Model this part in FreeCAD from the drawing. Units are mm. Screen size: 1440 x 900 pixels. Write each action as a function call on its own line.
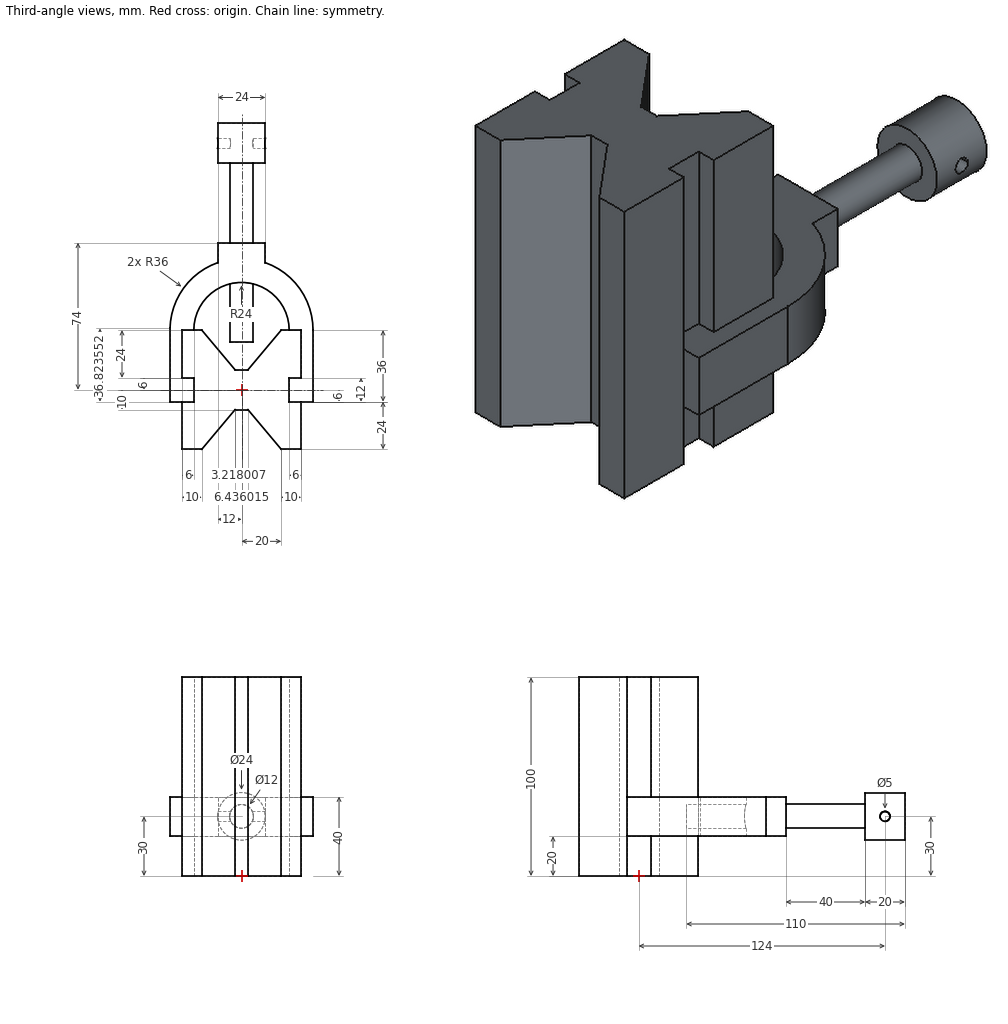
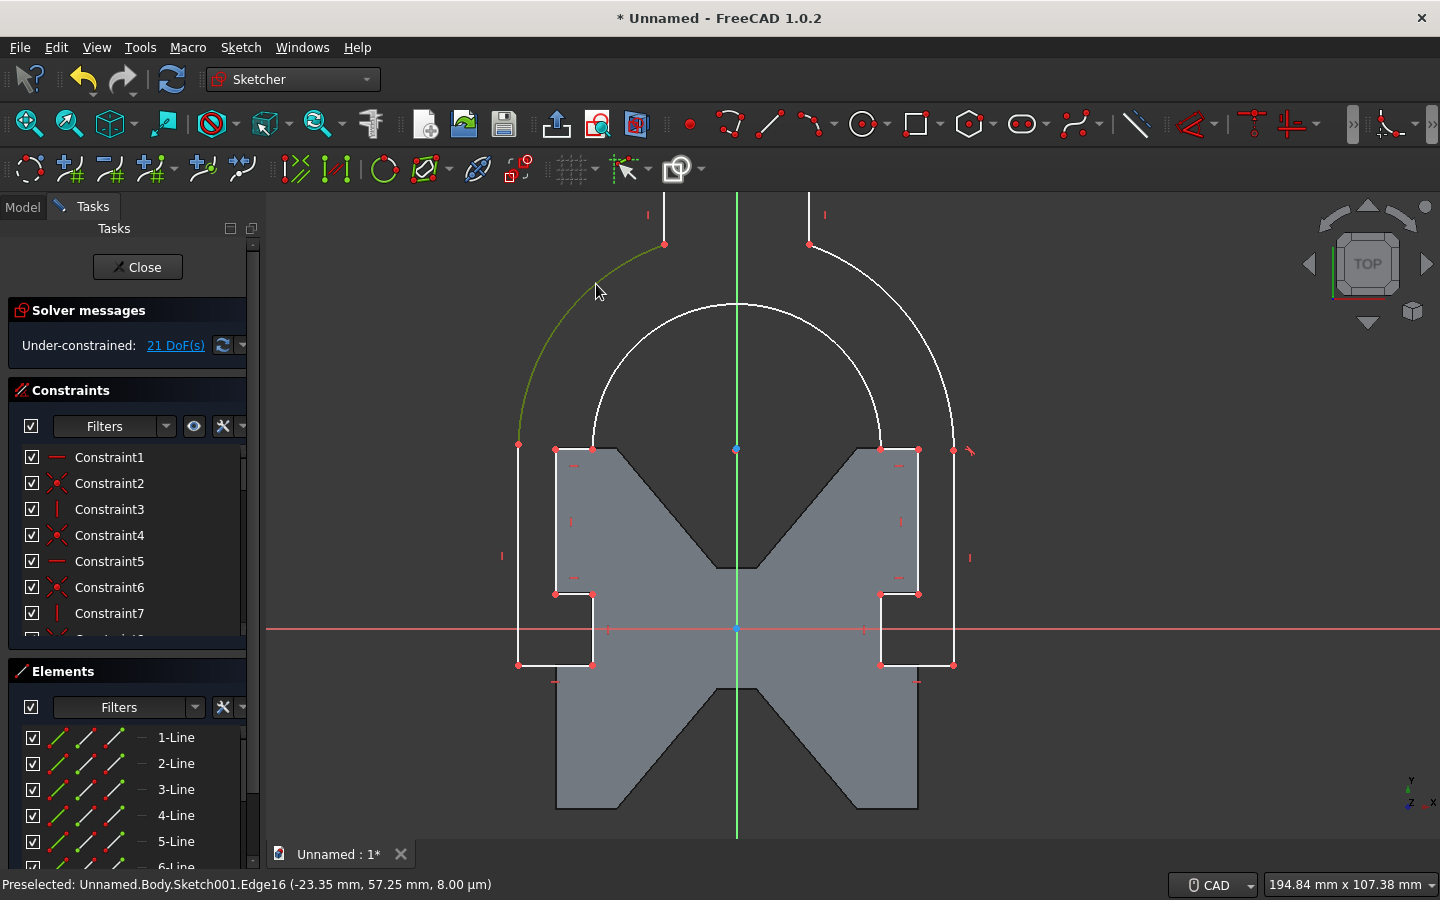
click(822, 332)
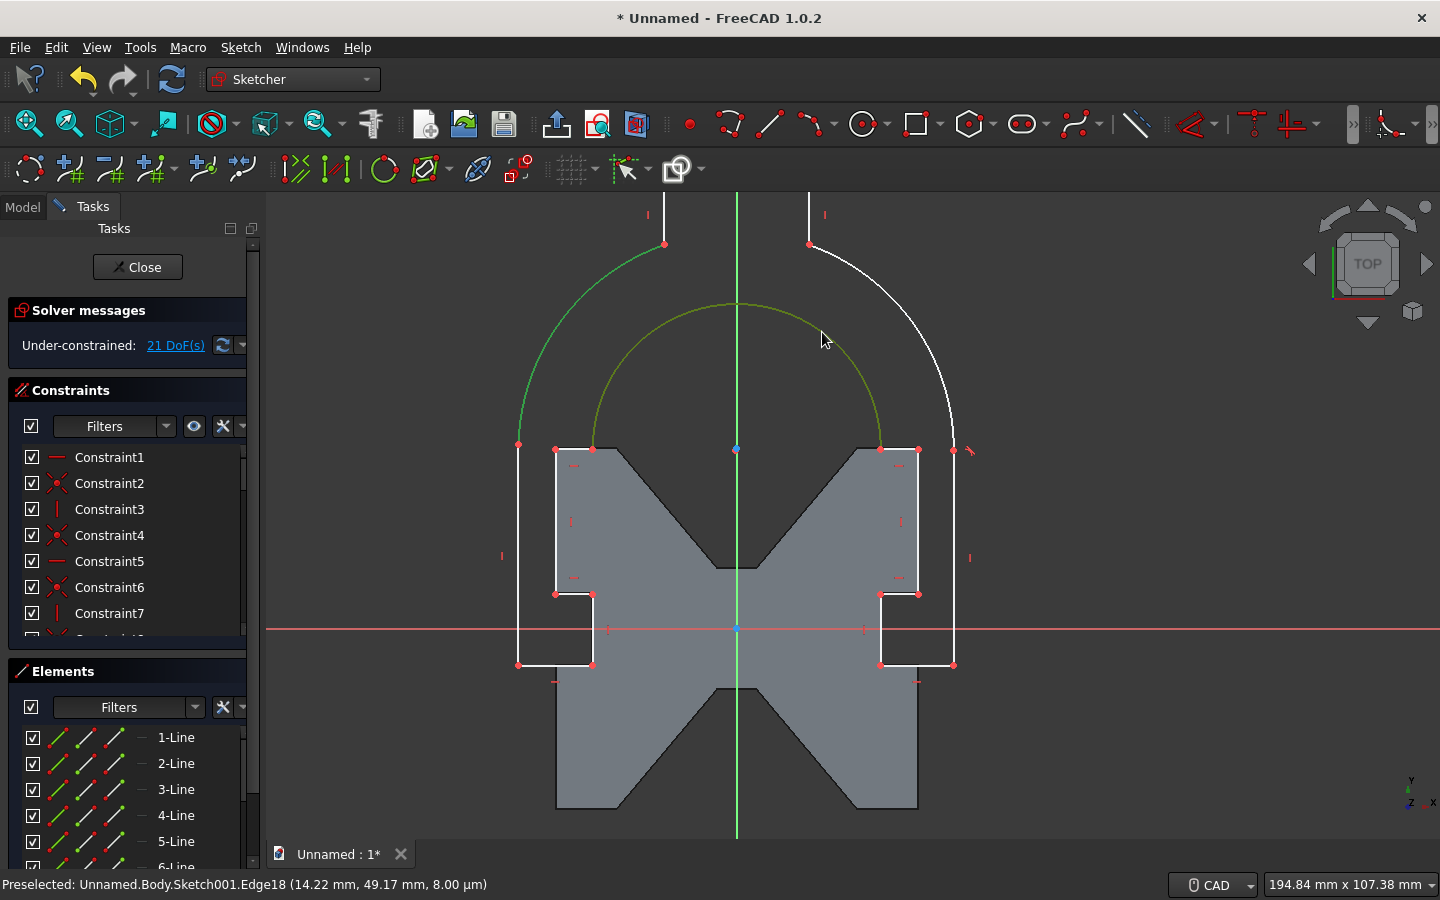
click(1252, 124)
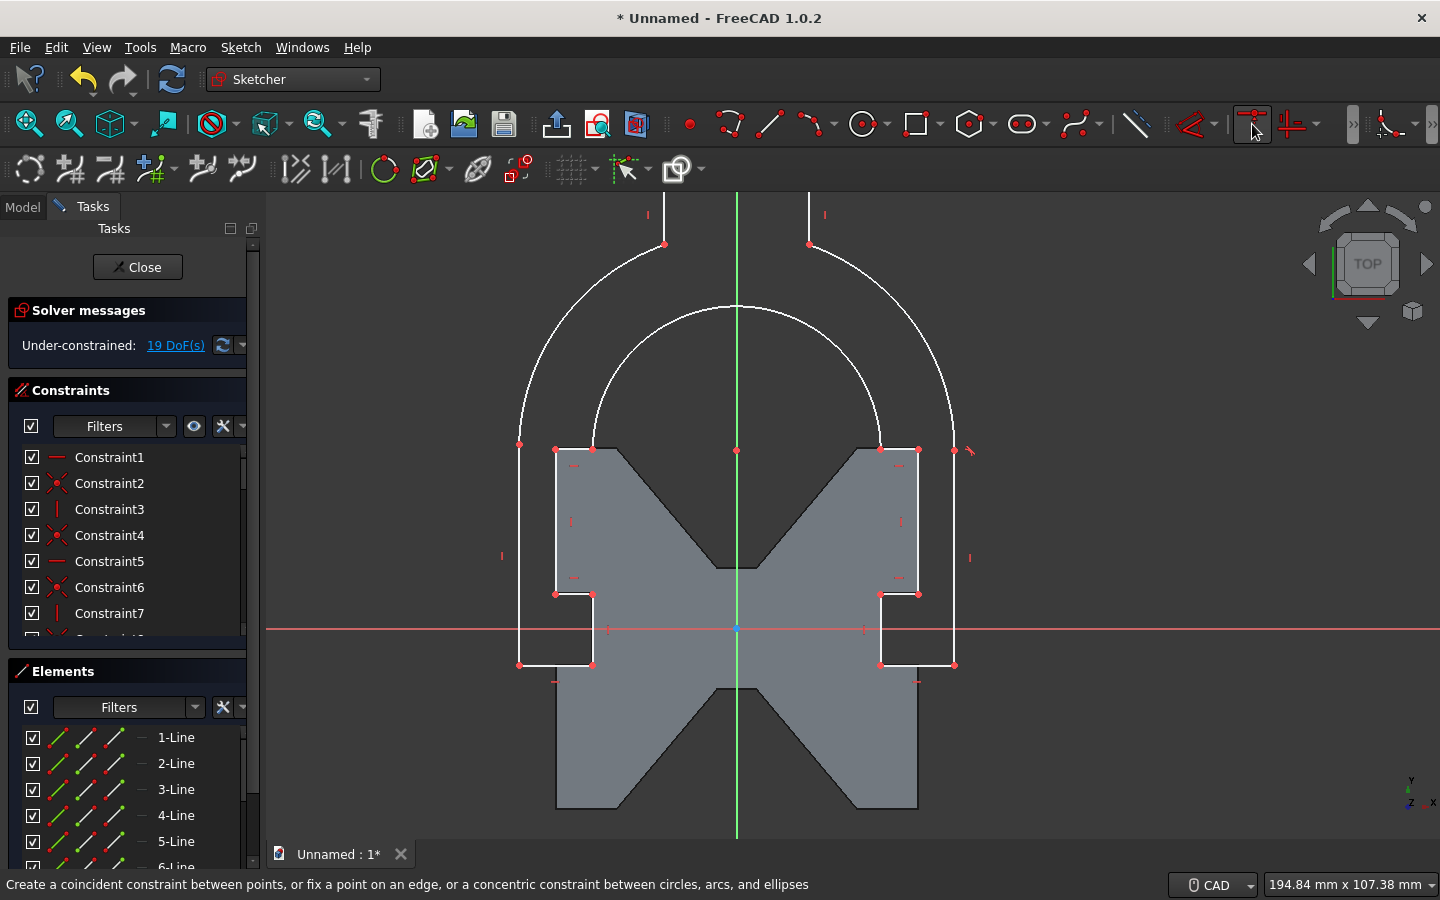
click(596, 284)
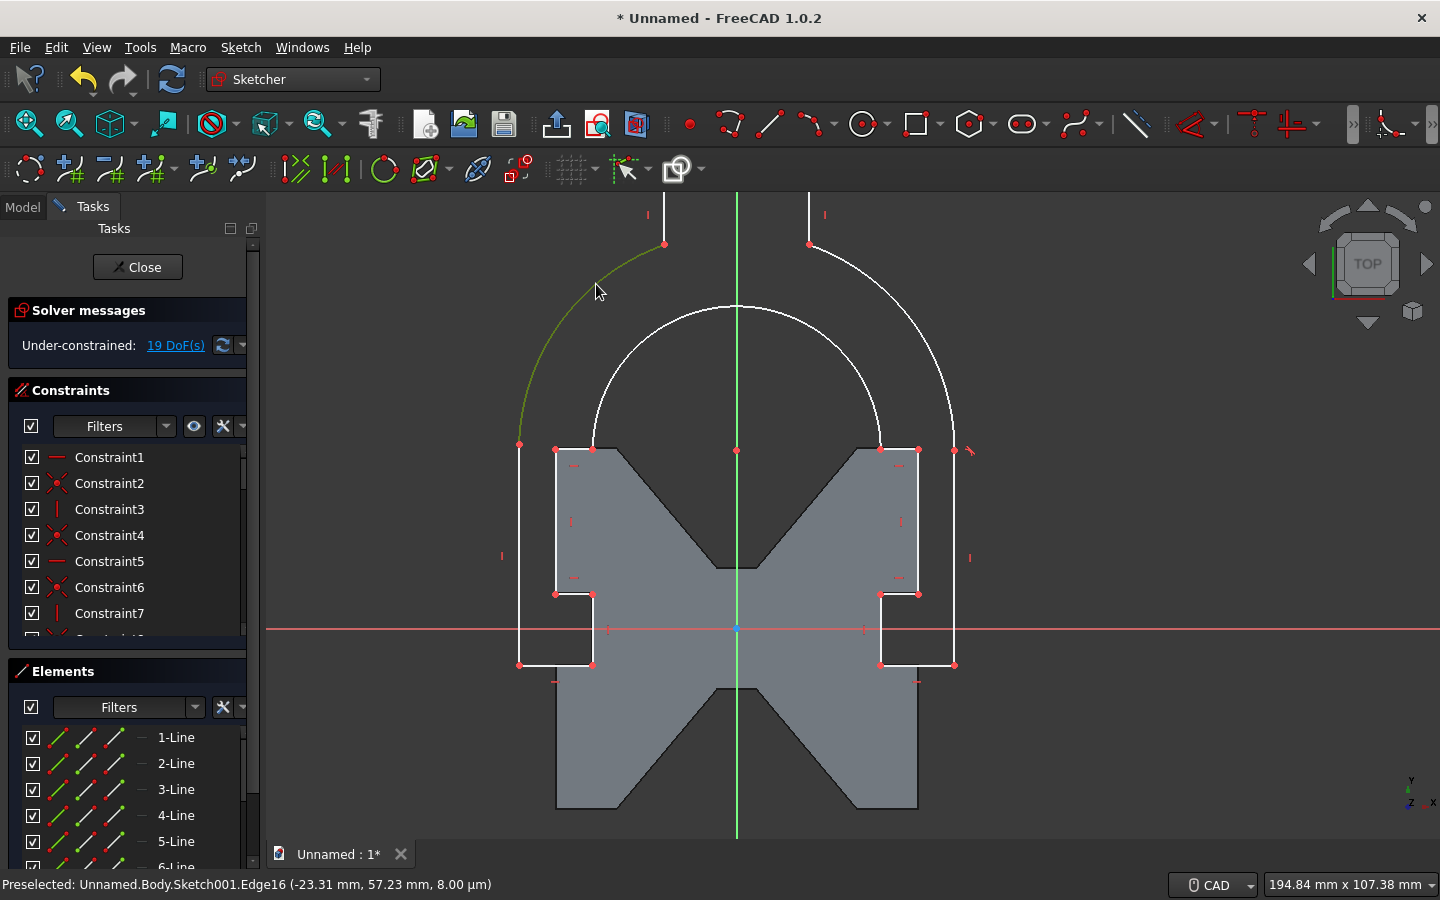
click(940, 372)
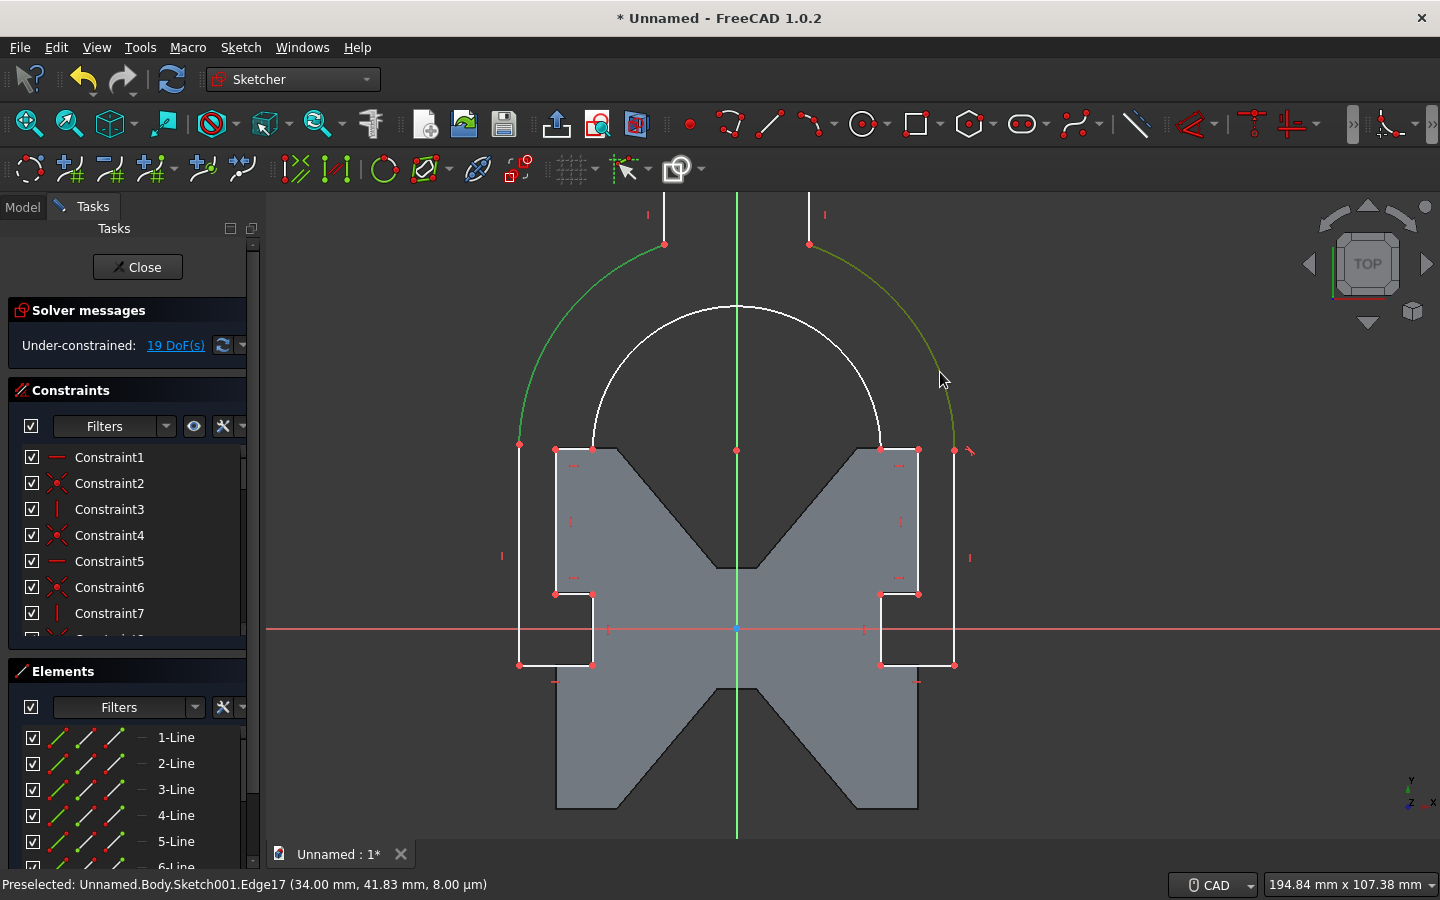
key(e)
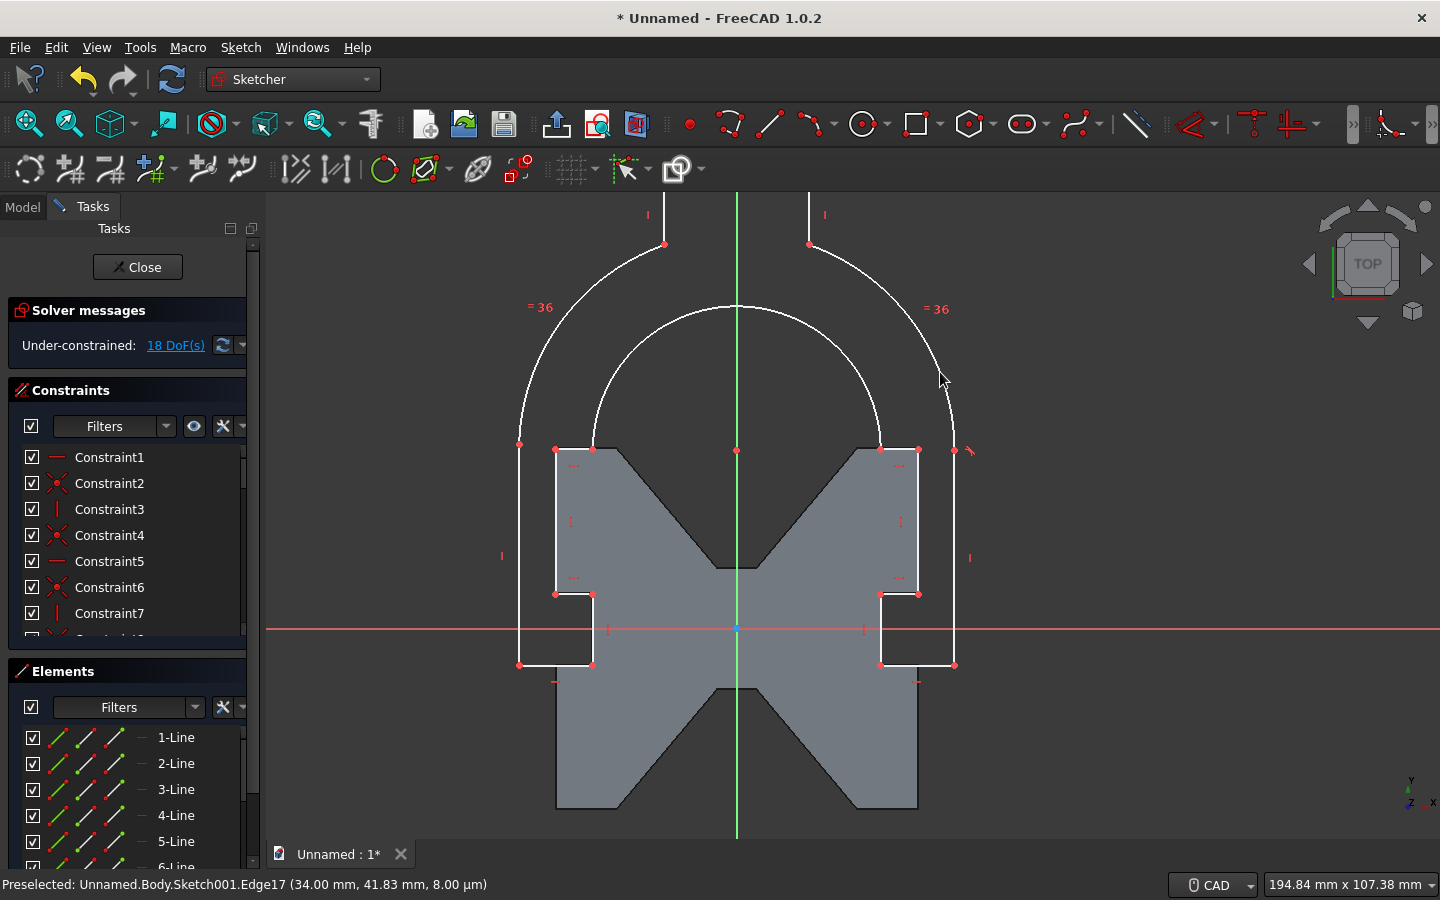
click(737, 450)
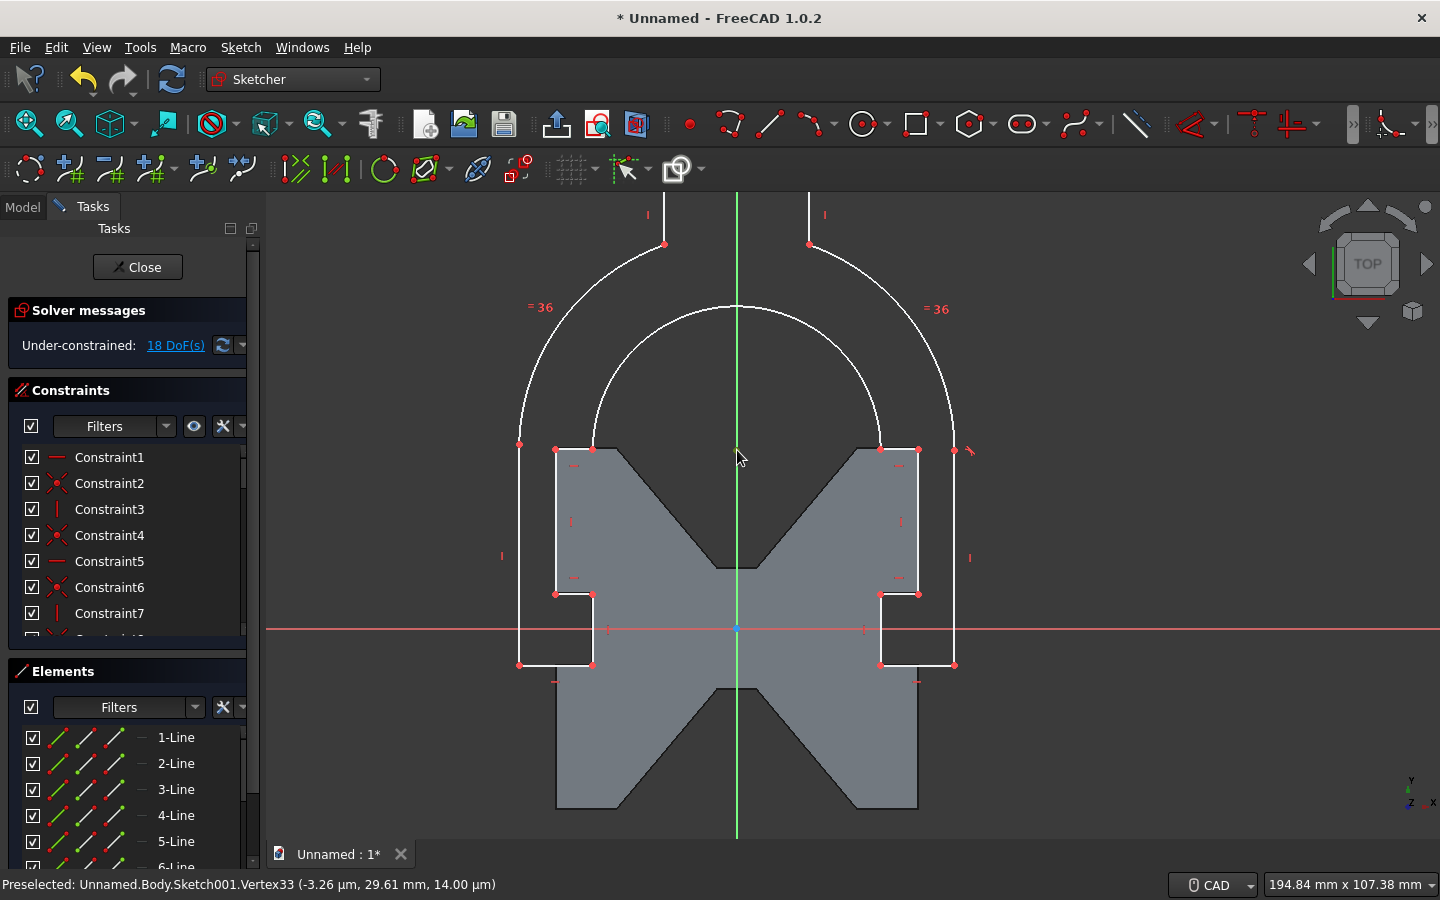
click(737, 769)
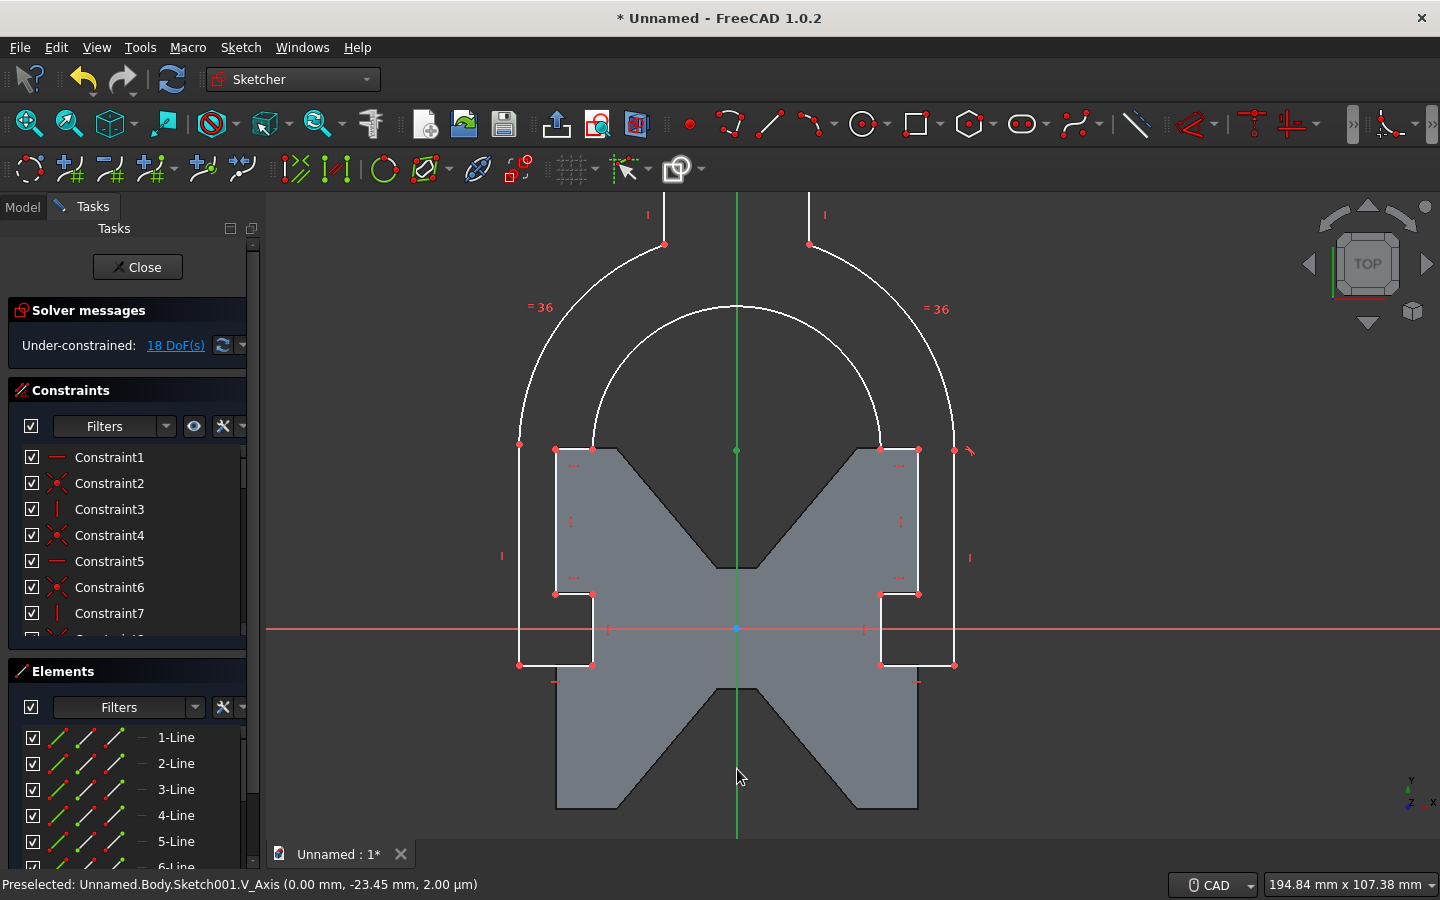
key(c)